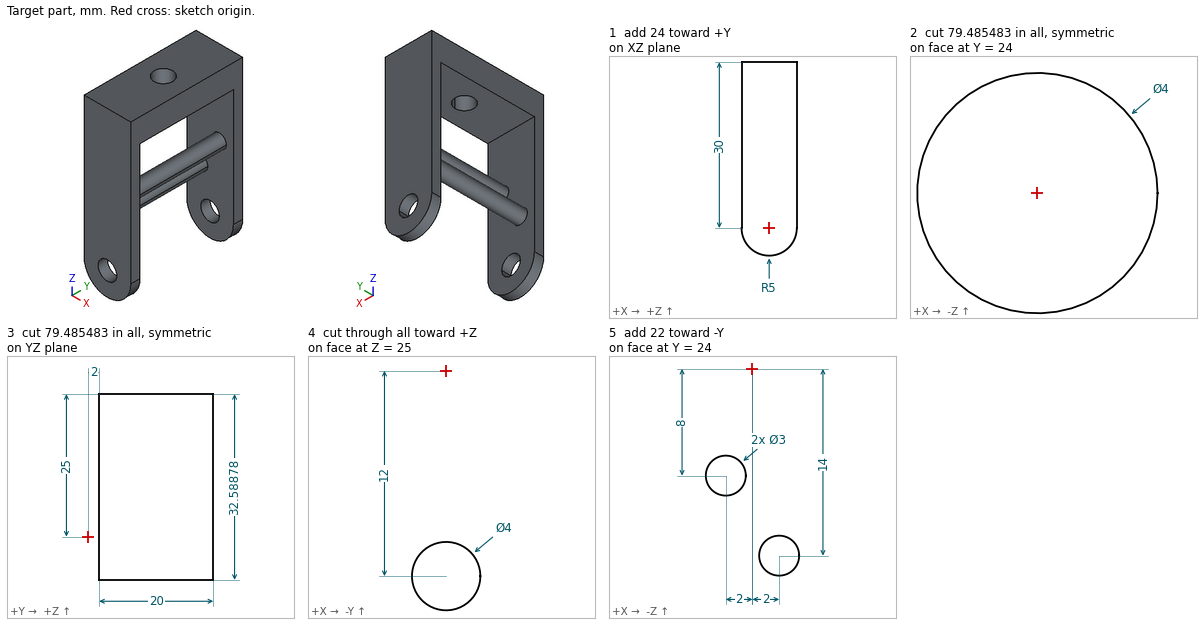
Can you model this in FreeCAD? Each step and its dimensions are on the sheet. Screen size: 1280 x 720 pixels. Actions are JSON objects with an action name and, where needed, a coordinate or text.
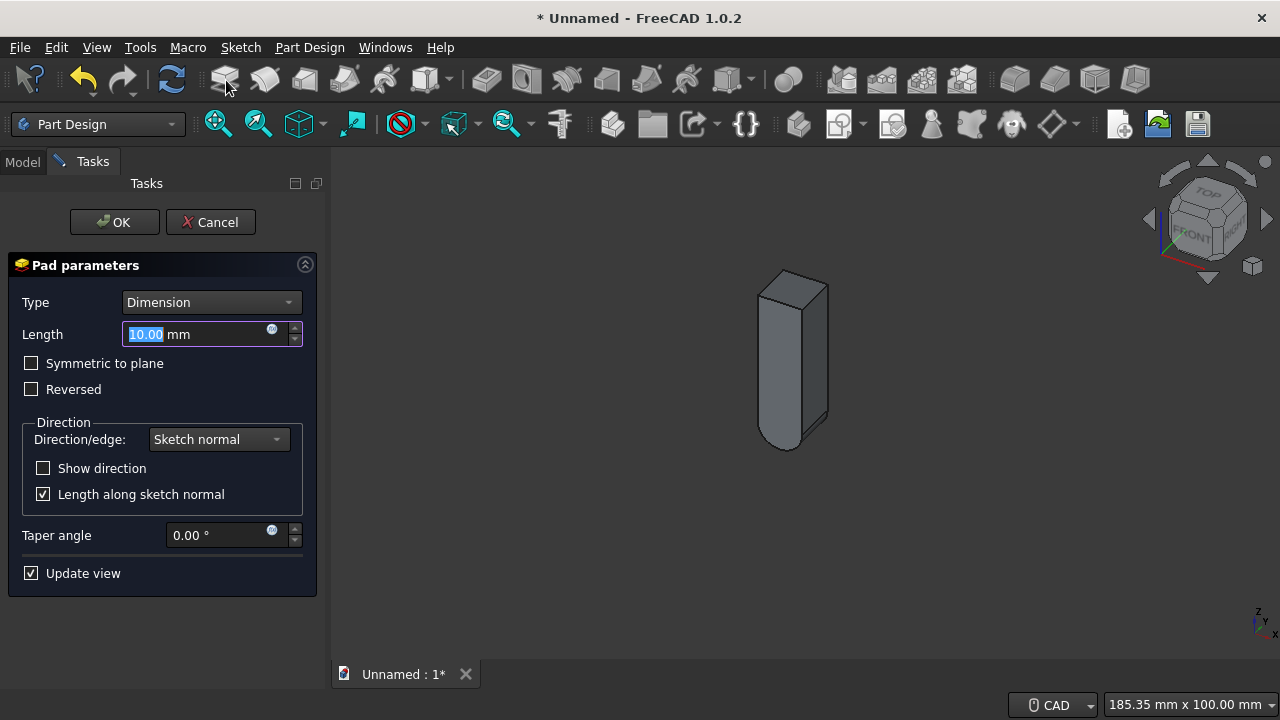
{"action": "type", "text": "24"}
{"action": "key", "text": "Tab"}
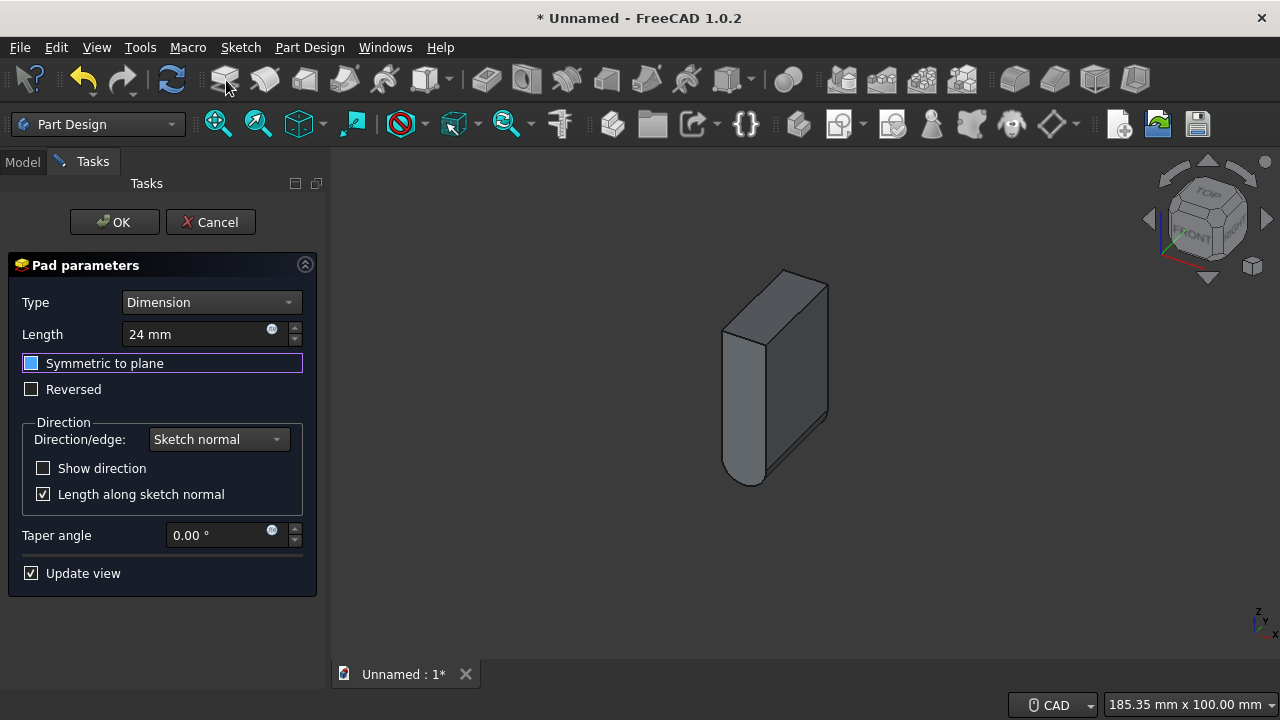
{"action": "left_click", "coordinate": [30, 389]}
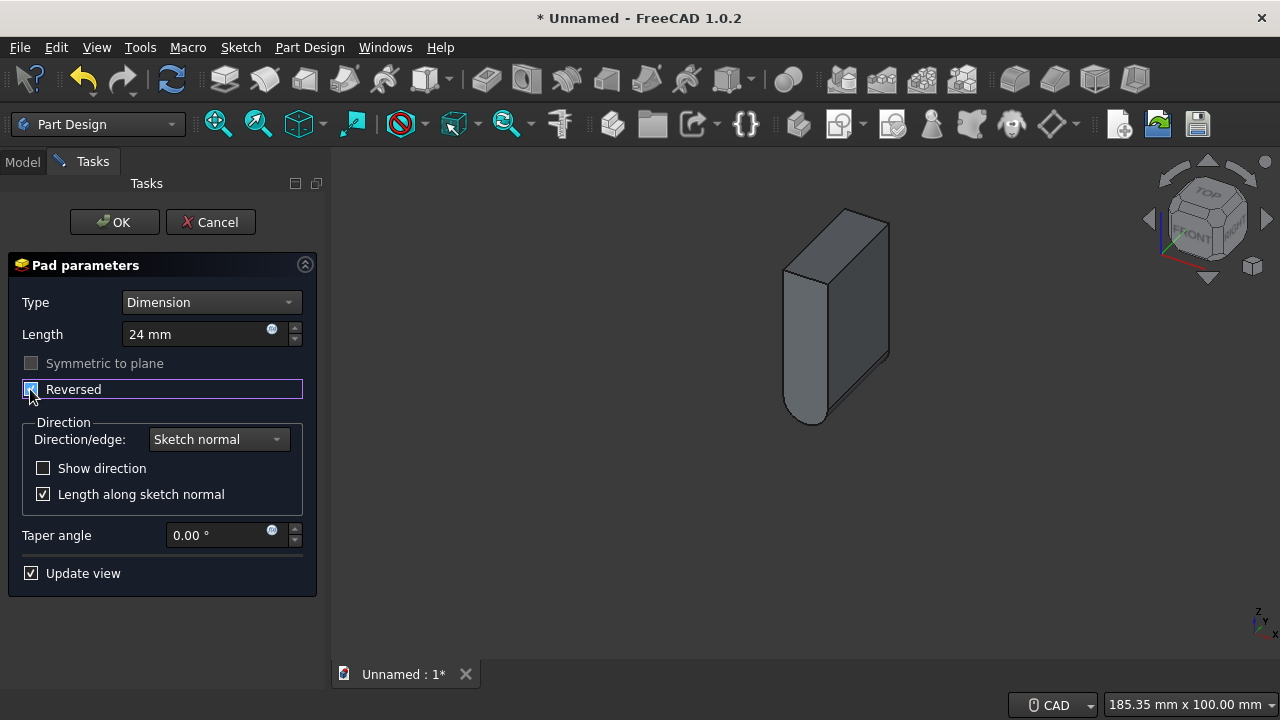
{"action": "left_click", "coordinate": [115, 222]}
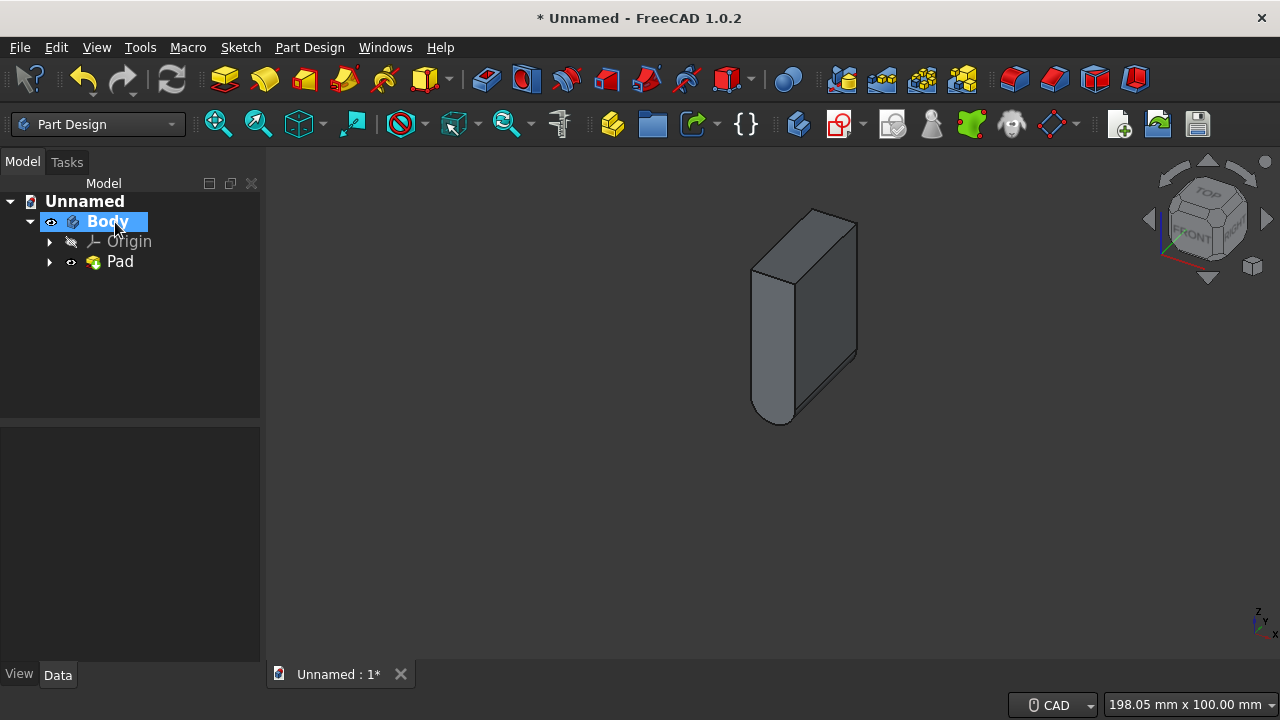
{"action": "left_click", "coordinate": [220, 124]}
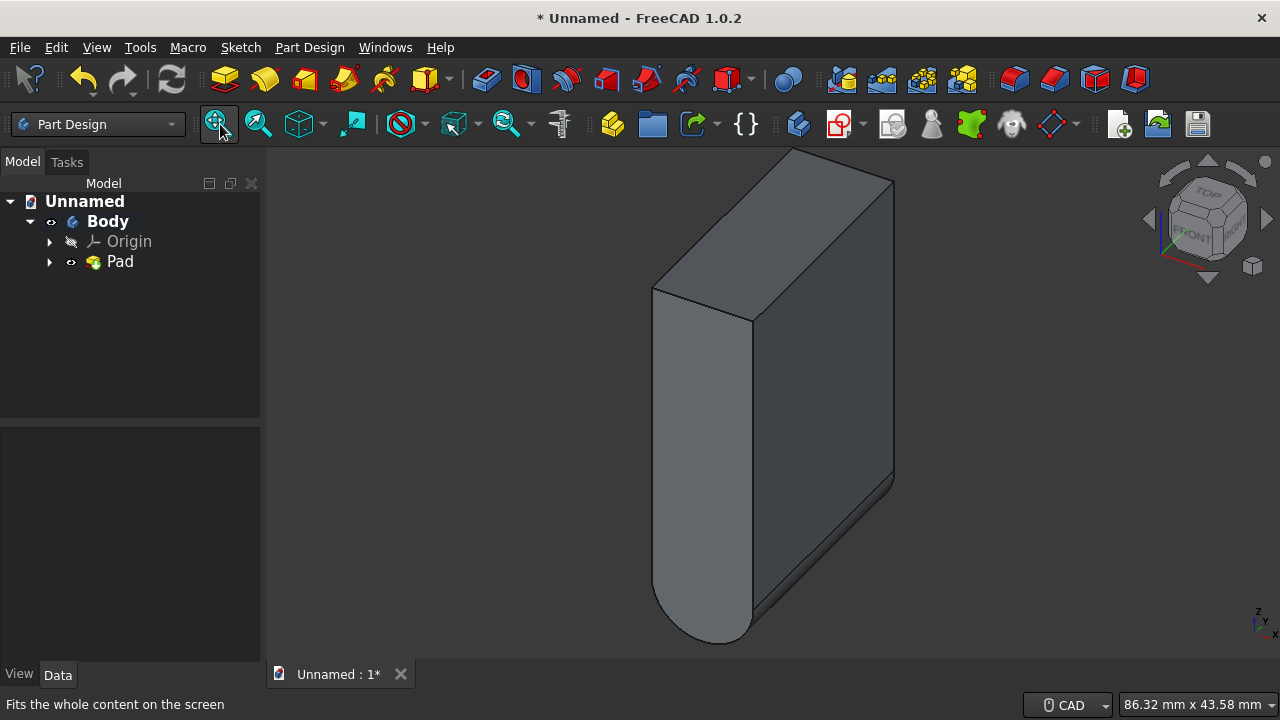
{"action": "key", "text": "4"}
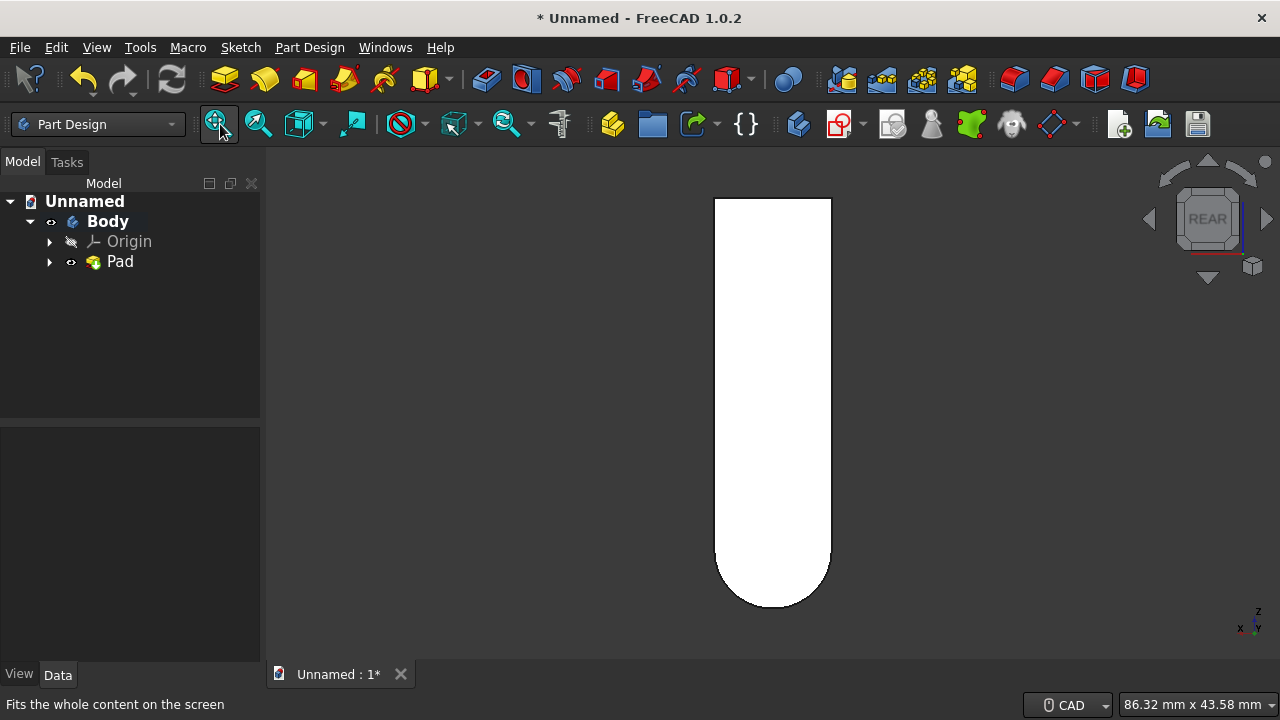
{"action": "left_click", "coordinate": [773, 285]}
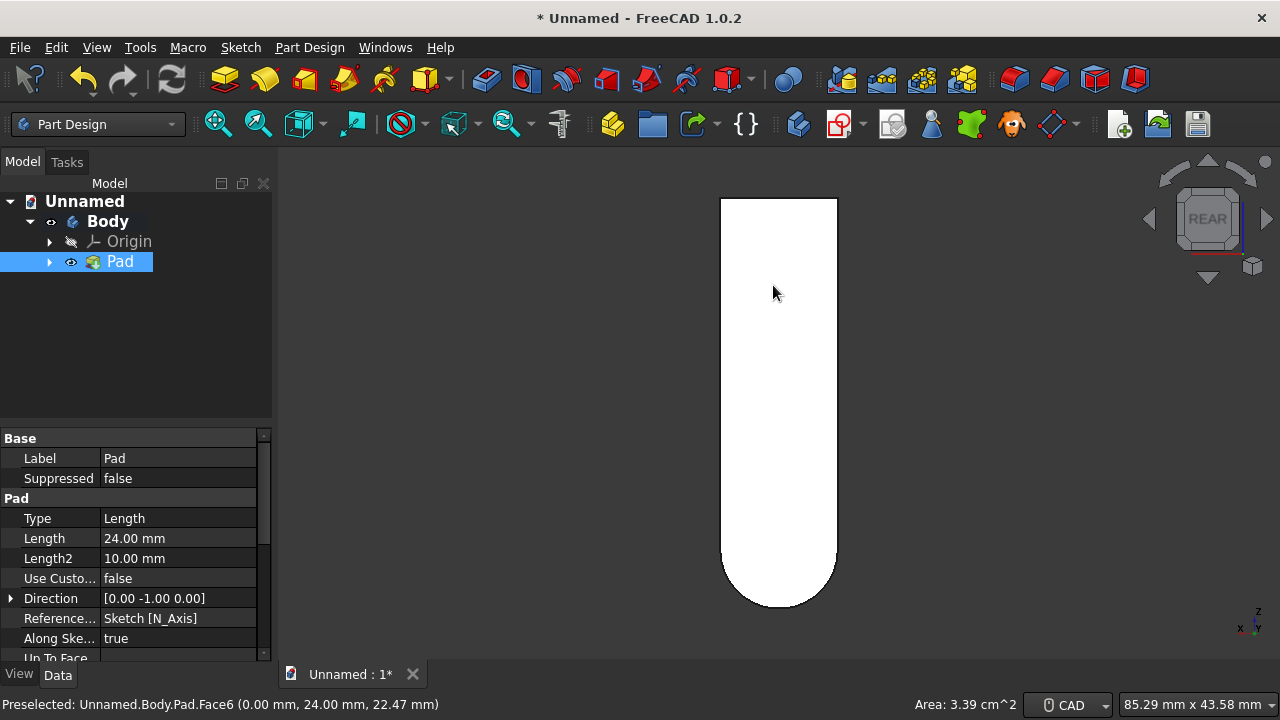
{"action": "left_click", "coordinate": [840, 124]}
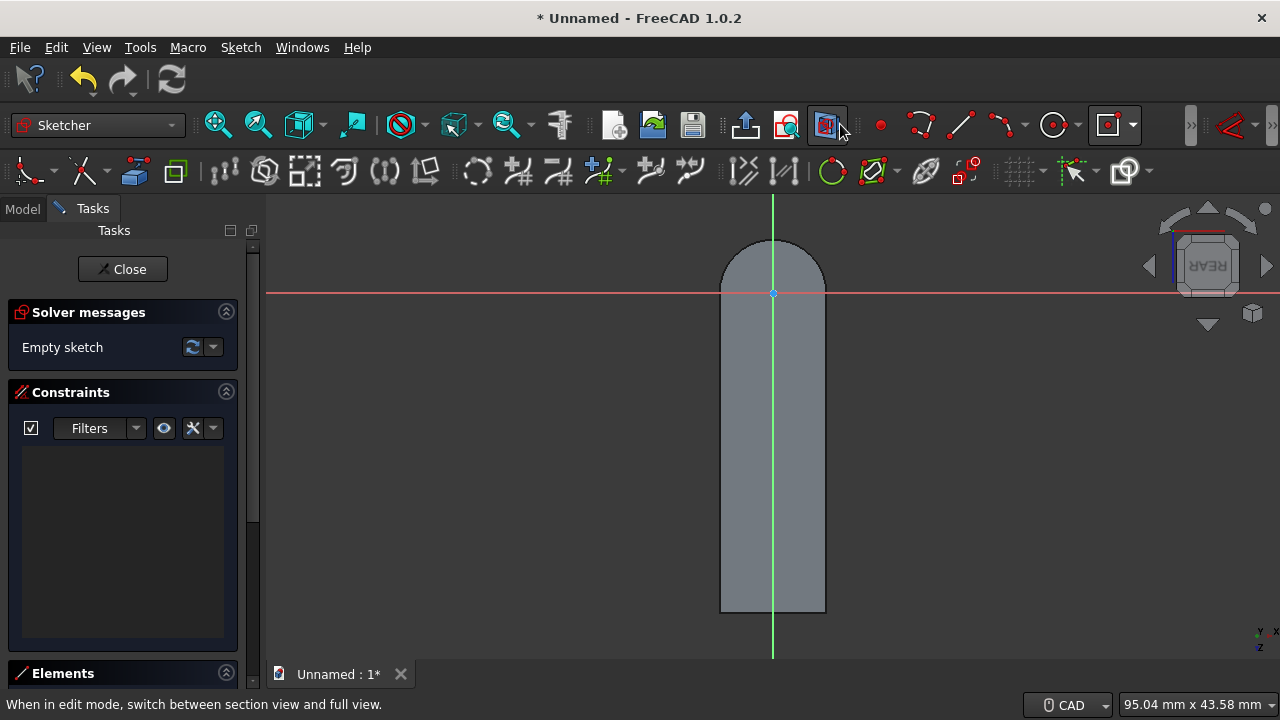
{"action": "scroll", "coordinate": [784, 272], "scroll_direction": "up", "scroll_amount": 10}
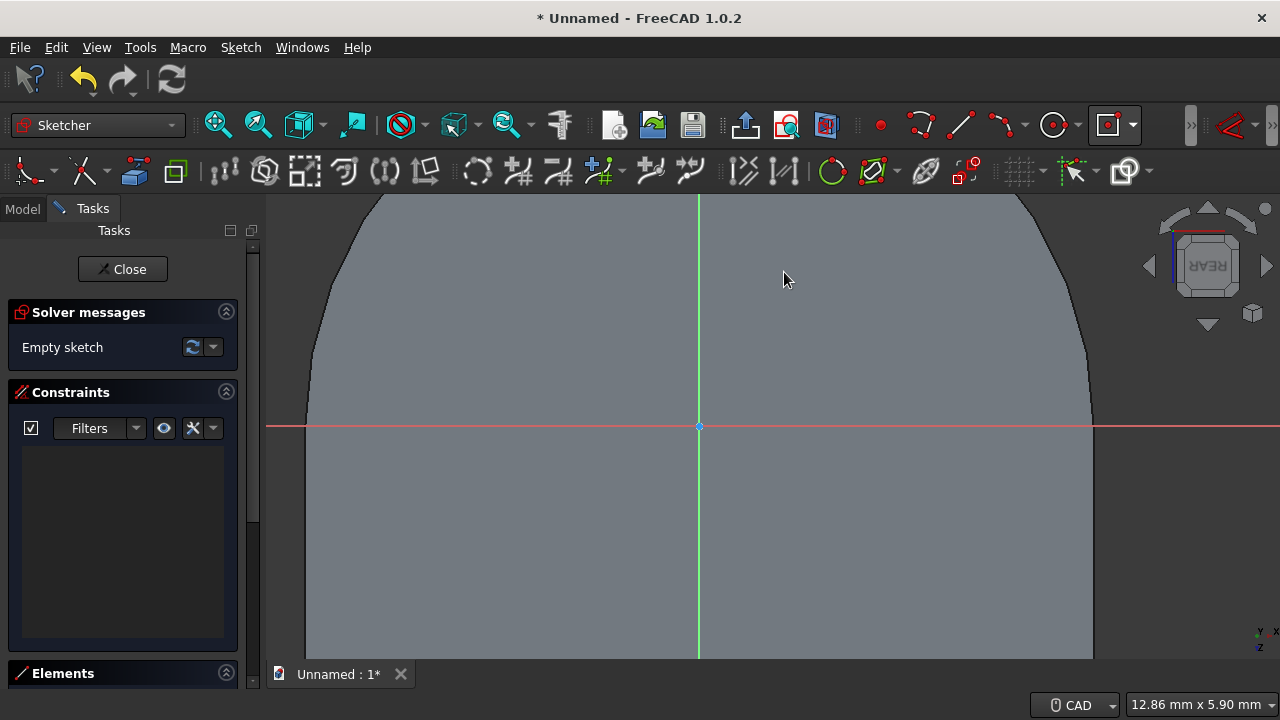
{"action": "left_click", "coordinate": [1054, 126]}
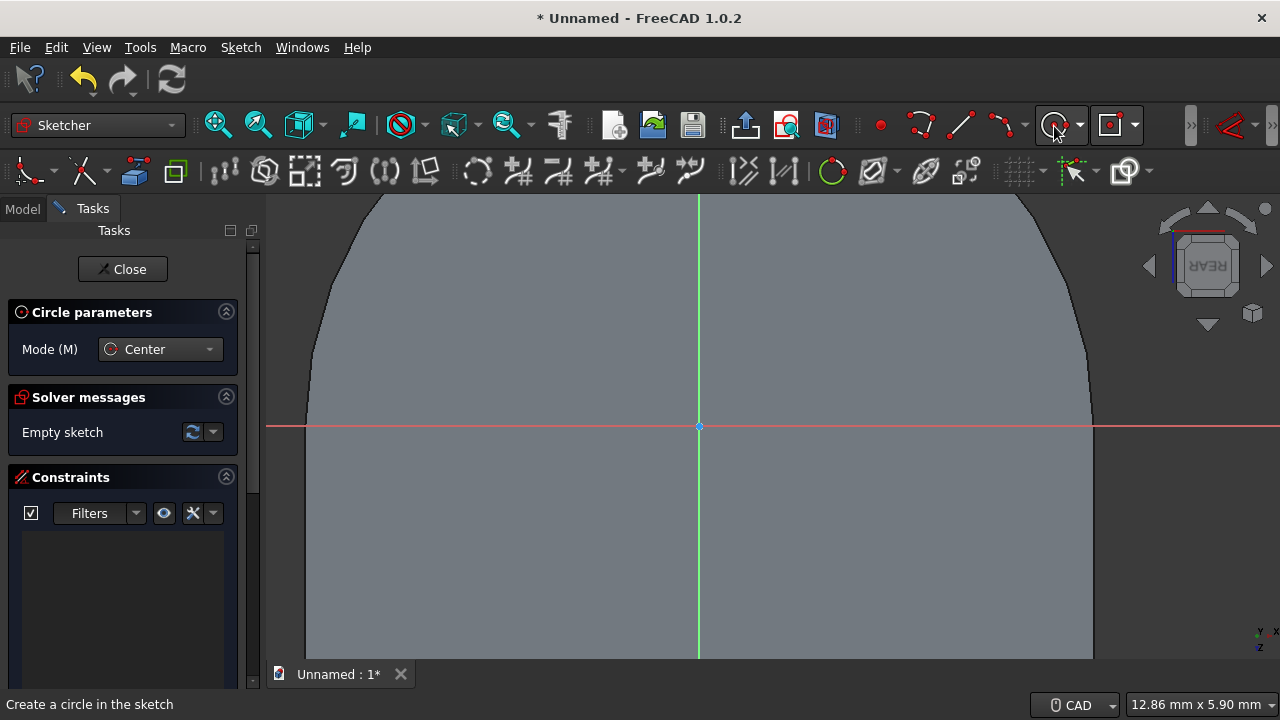
{"action": "left_click", "coordinate": [699, 426]}
{"action": "mouse_move", "coordinate": [811, 315]}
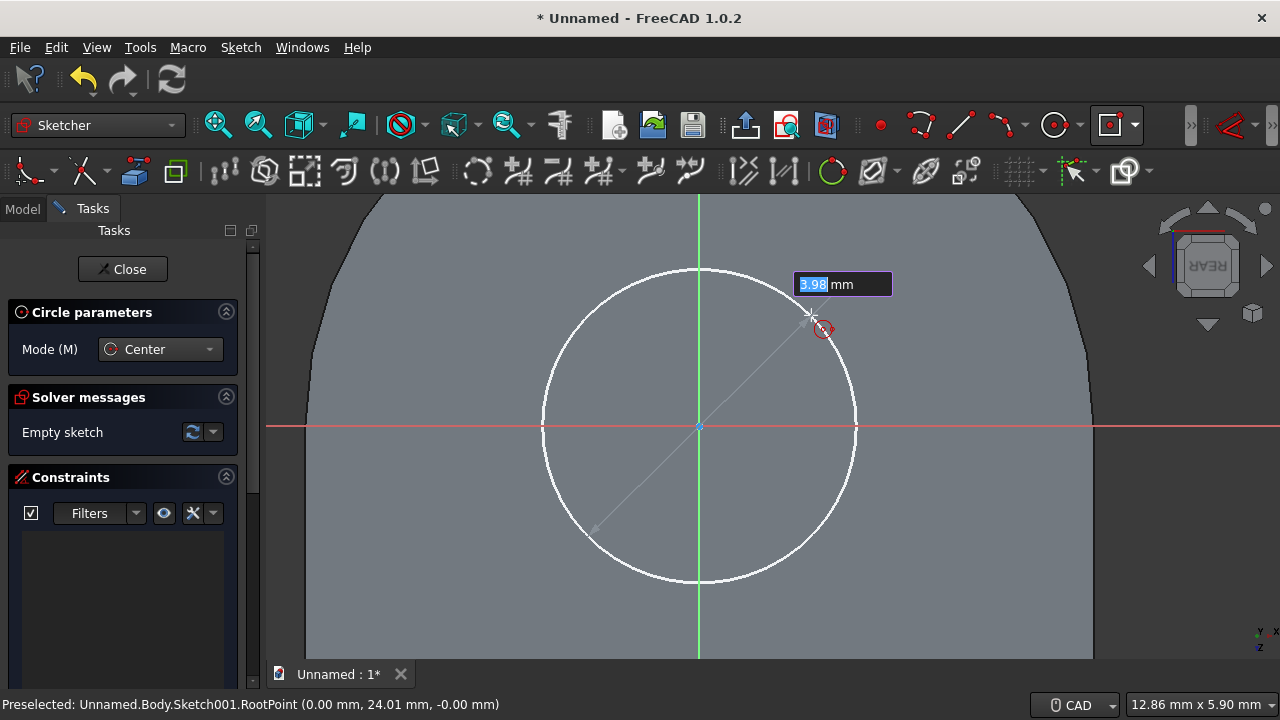
{"action": "type", "text": "4"}
{"action": "key", "text": "Return"}
{"action": "key", "text": "Escape"}